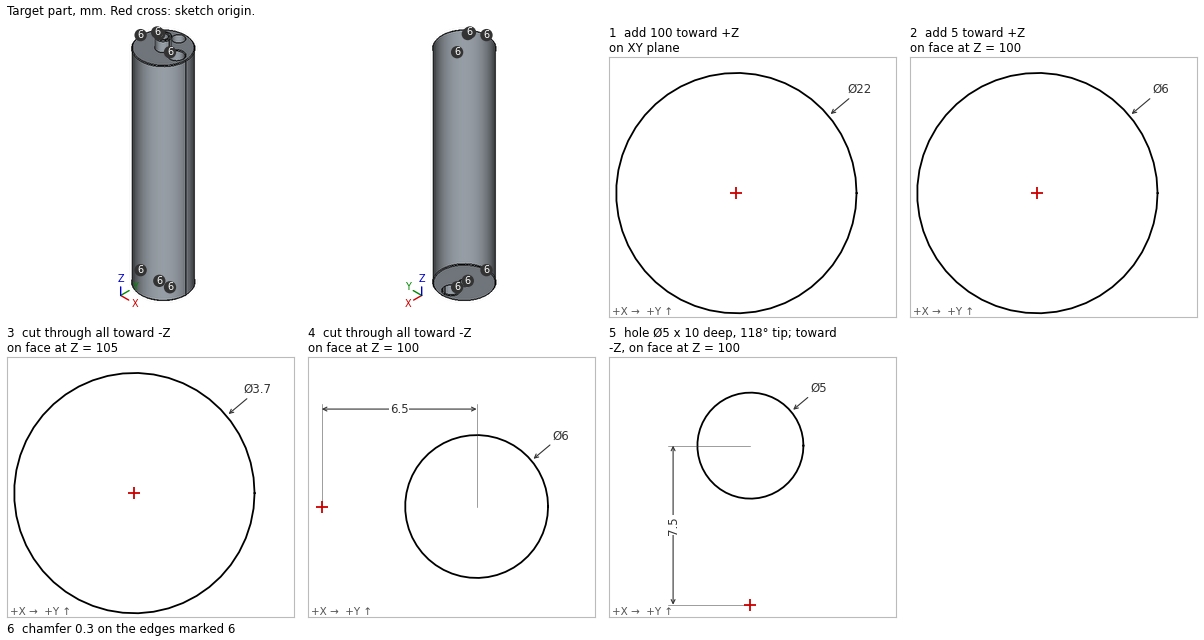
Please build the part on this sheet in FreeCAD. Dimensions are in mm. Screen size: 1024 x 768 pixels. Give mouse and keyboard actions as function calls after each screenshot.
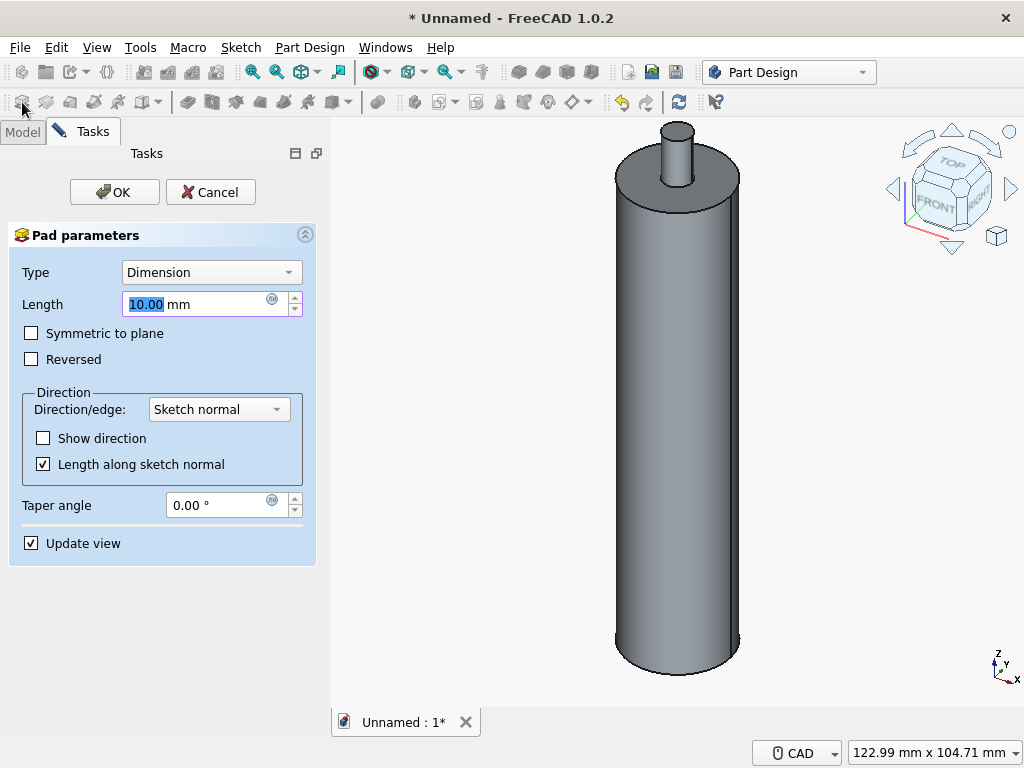
text(5)
key(Tab)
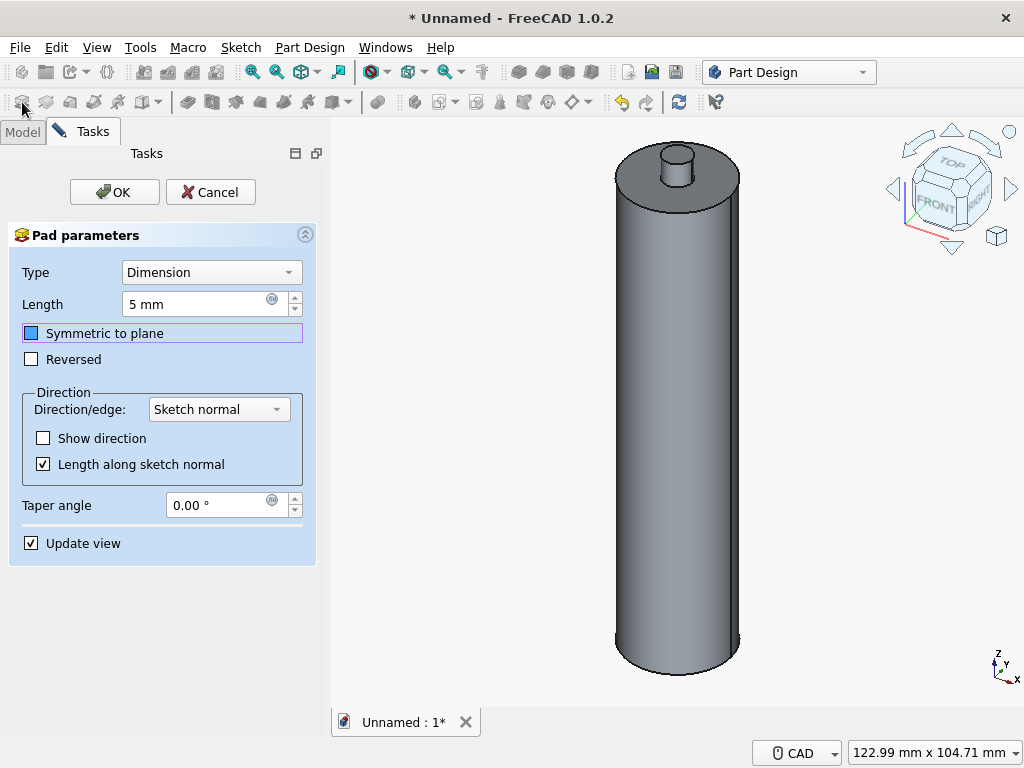
click(115, 192)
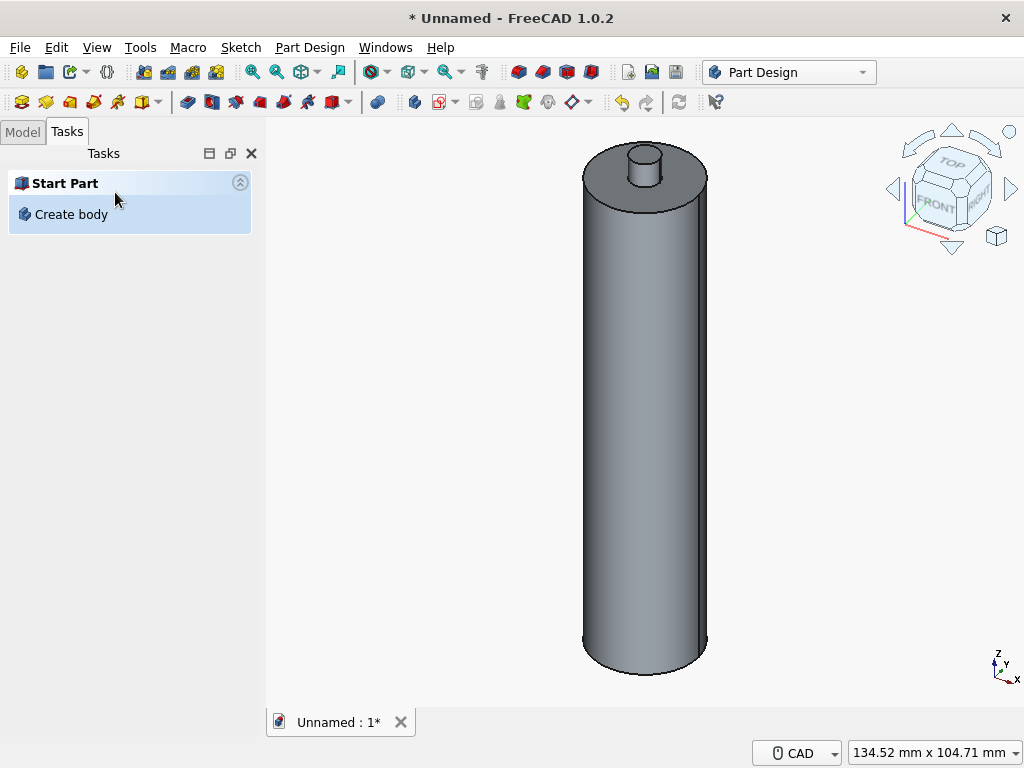
click(254, 72)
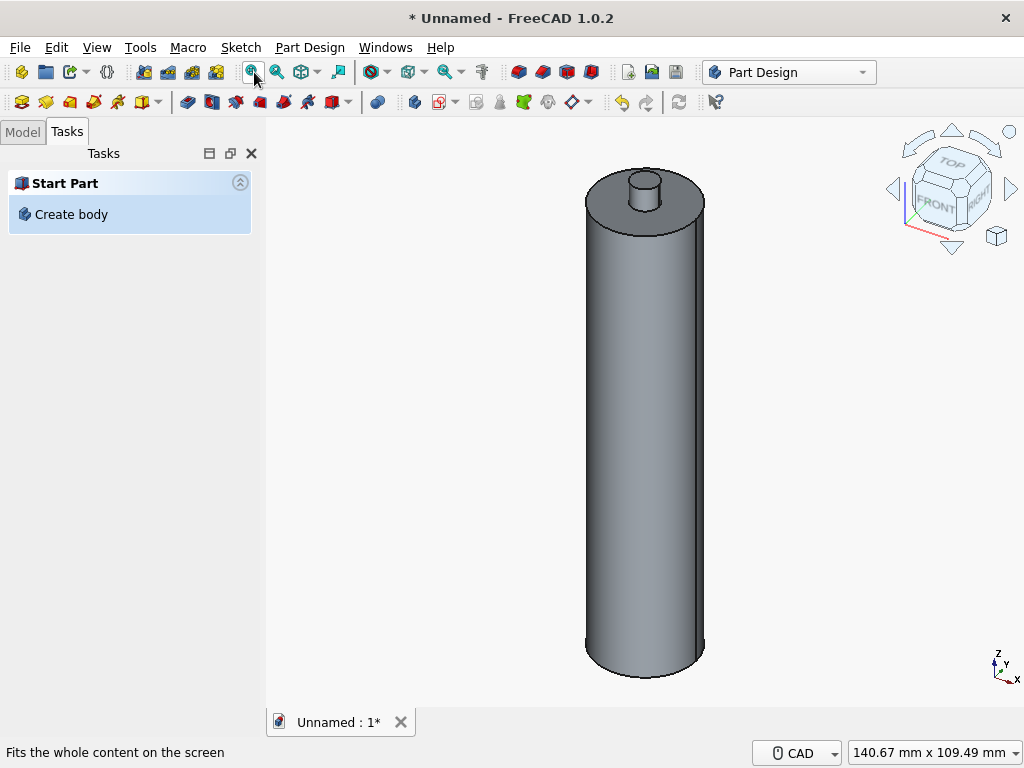
click(645, 179)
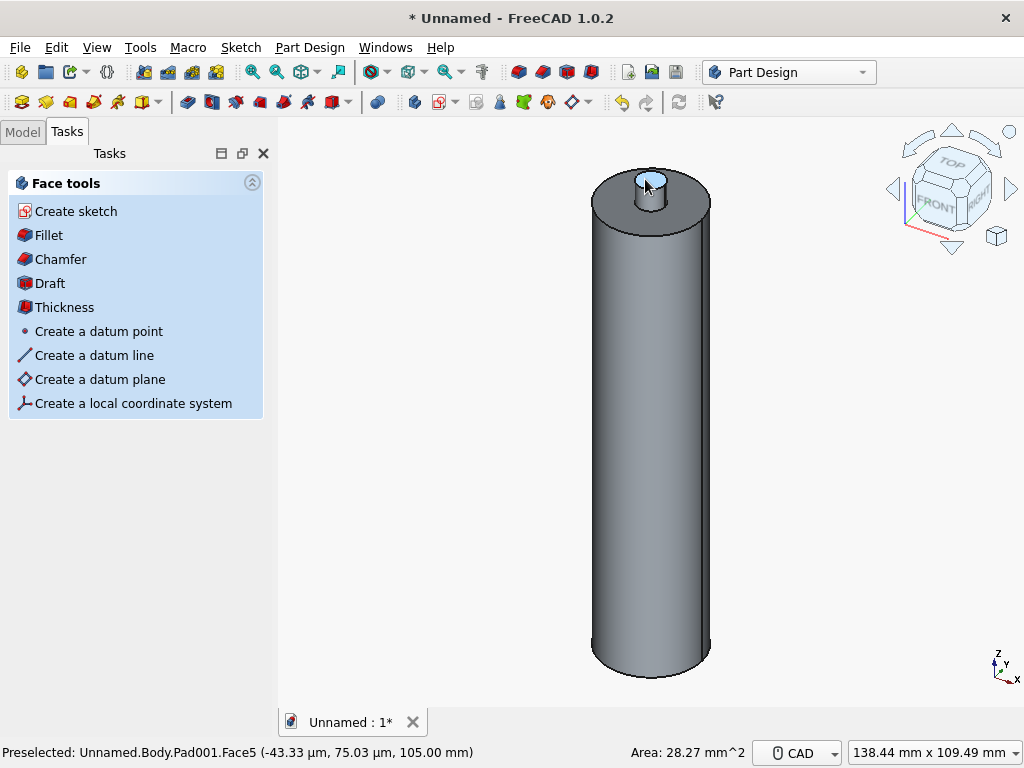
click(440, 102)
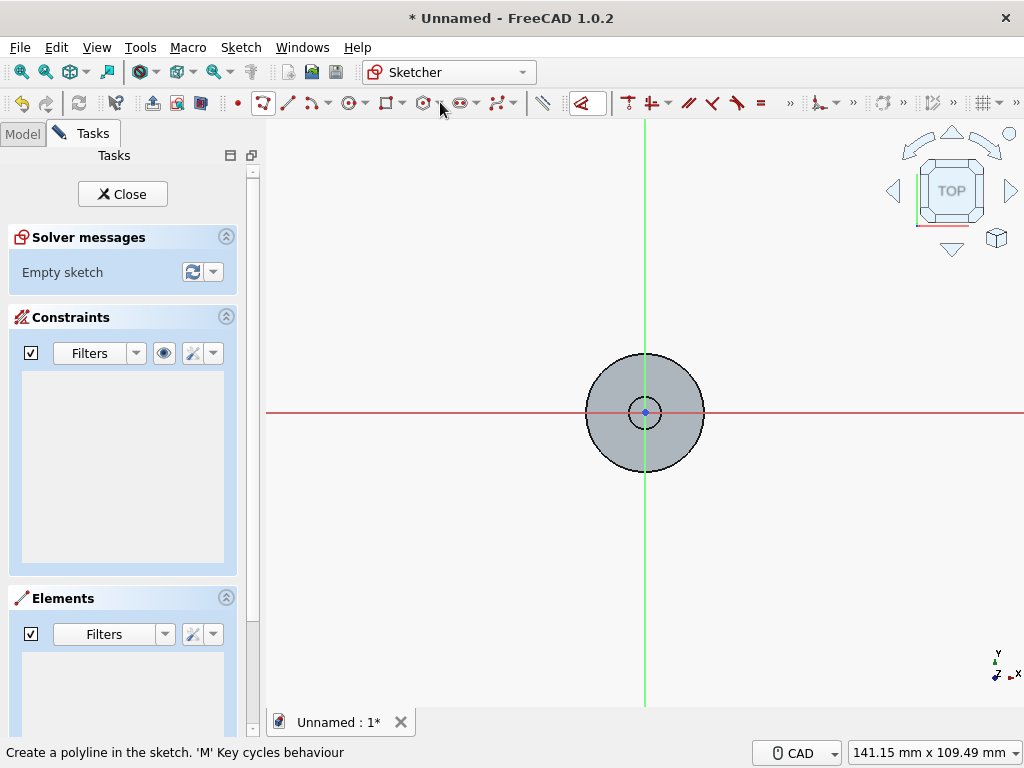
scroll(649, 413, up, 15)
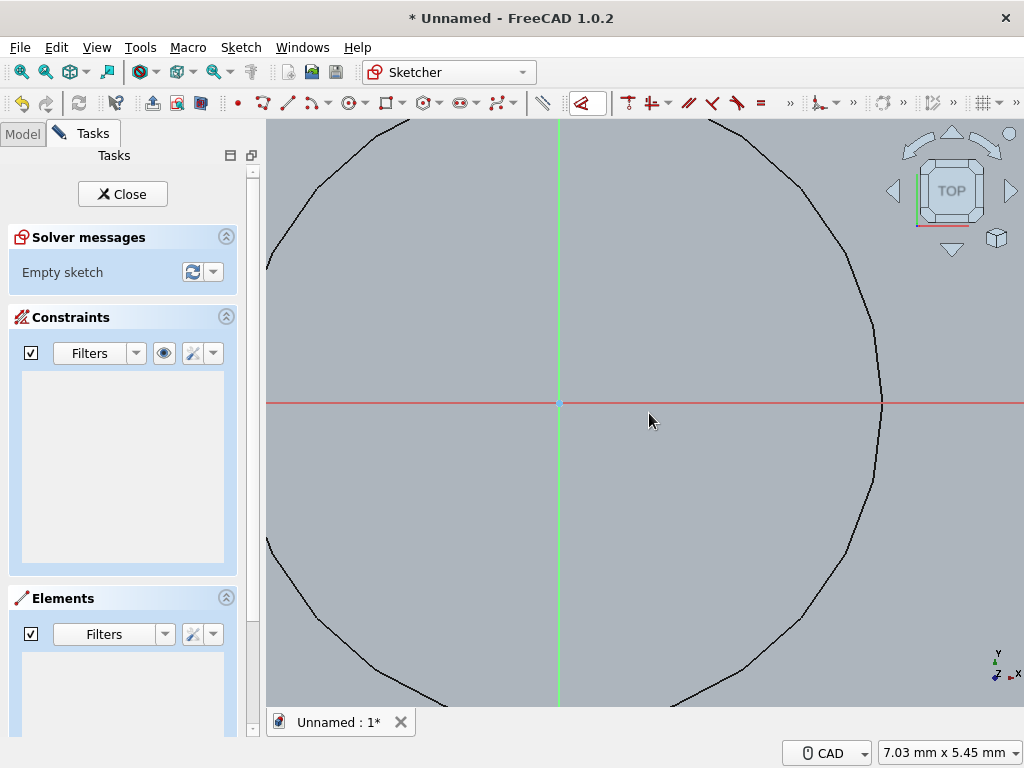
click(350, 104)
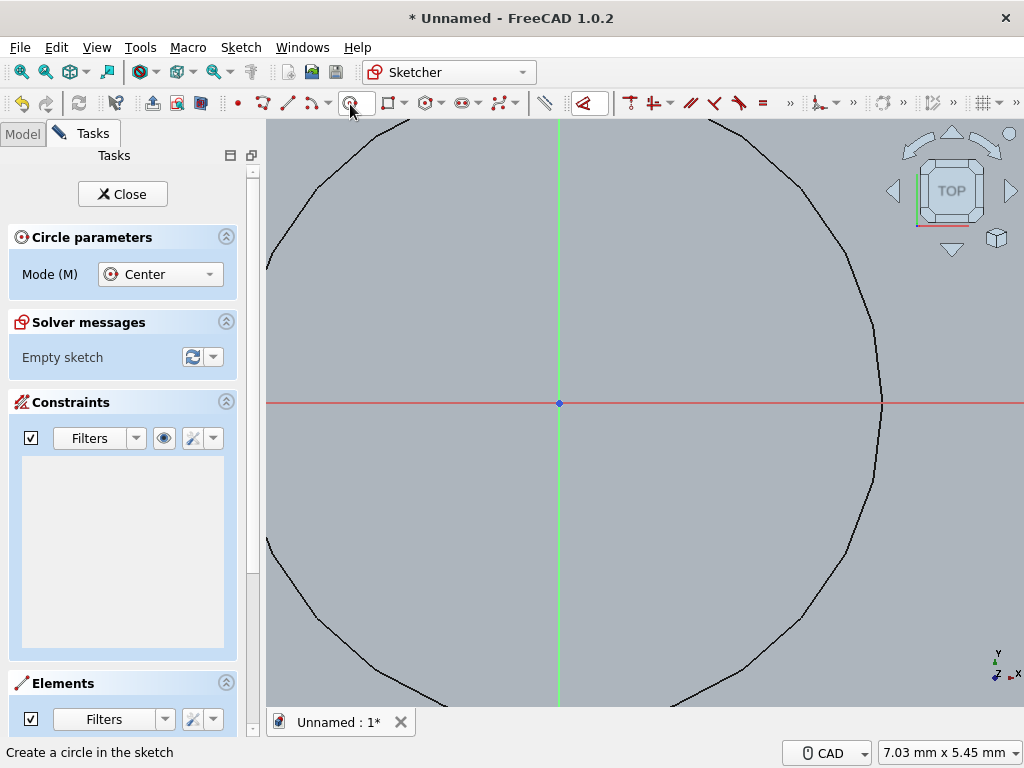
click(559, 403)
click(700, 262)
key(Escape)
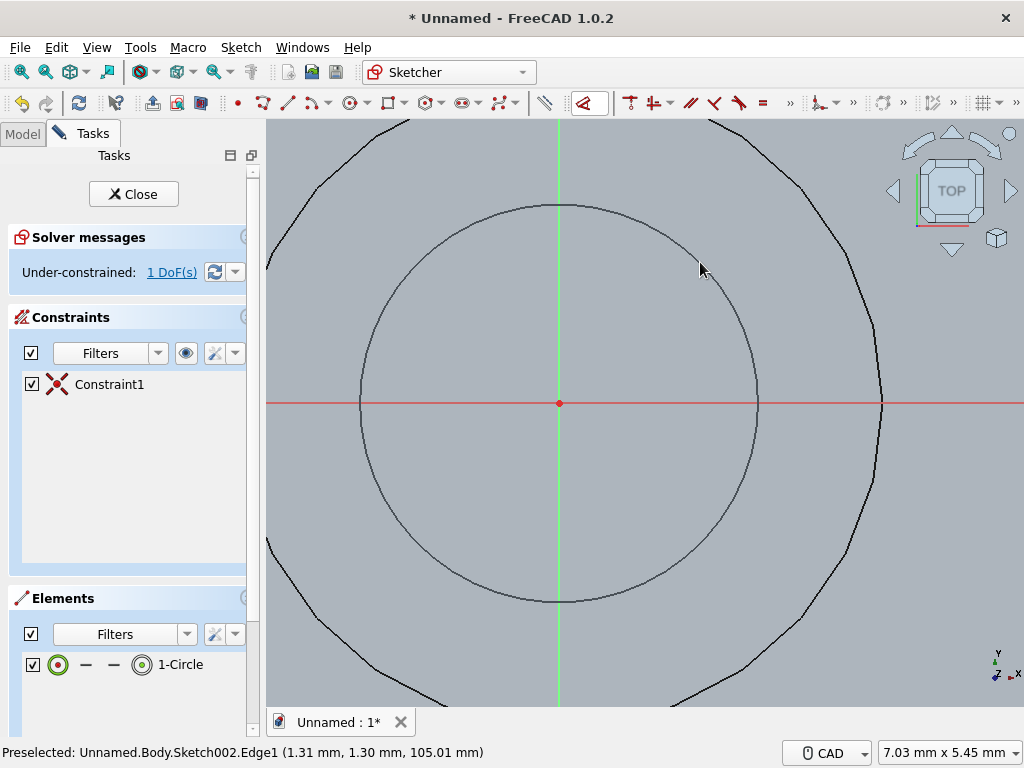
click(699, 262)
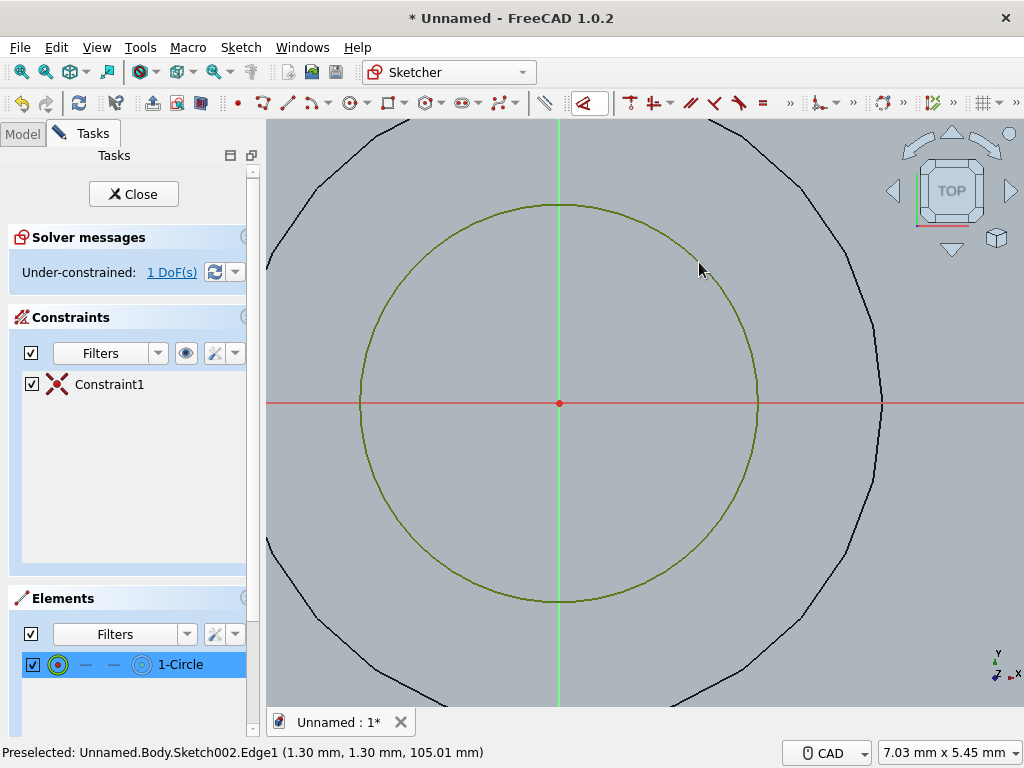
key(k)
key(o)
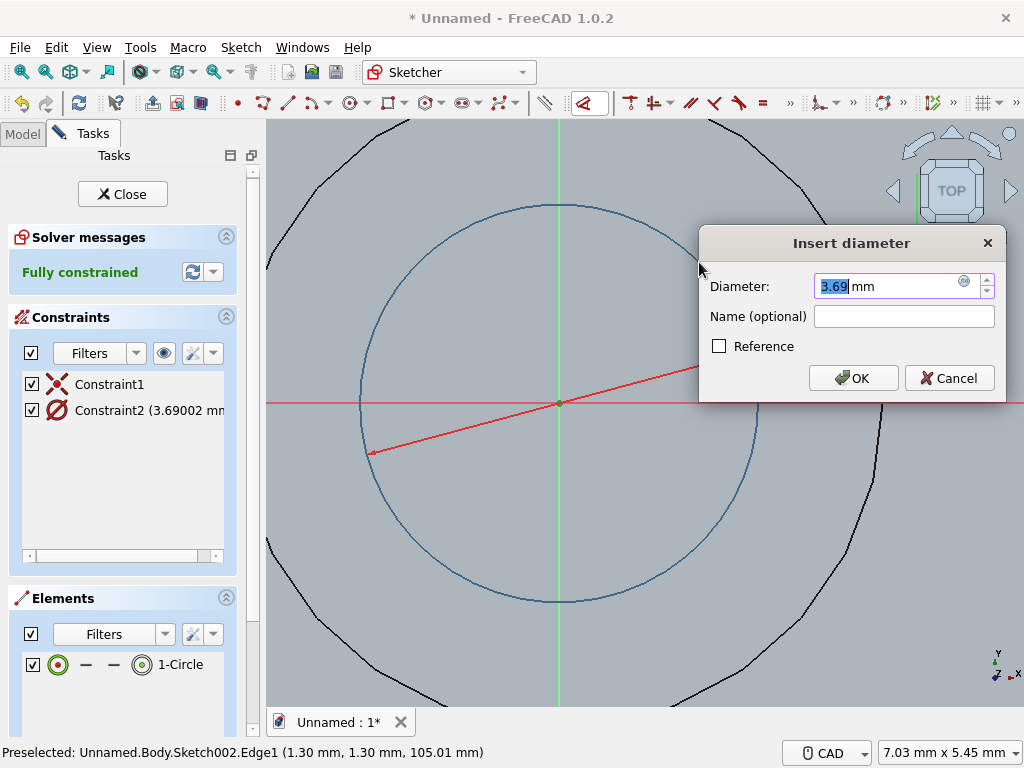
text(3.7)
key(Return)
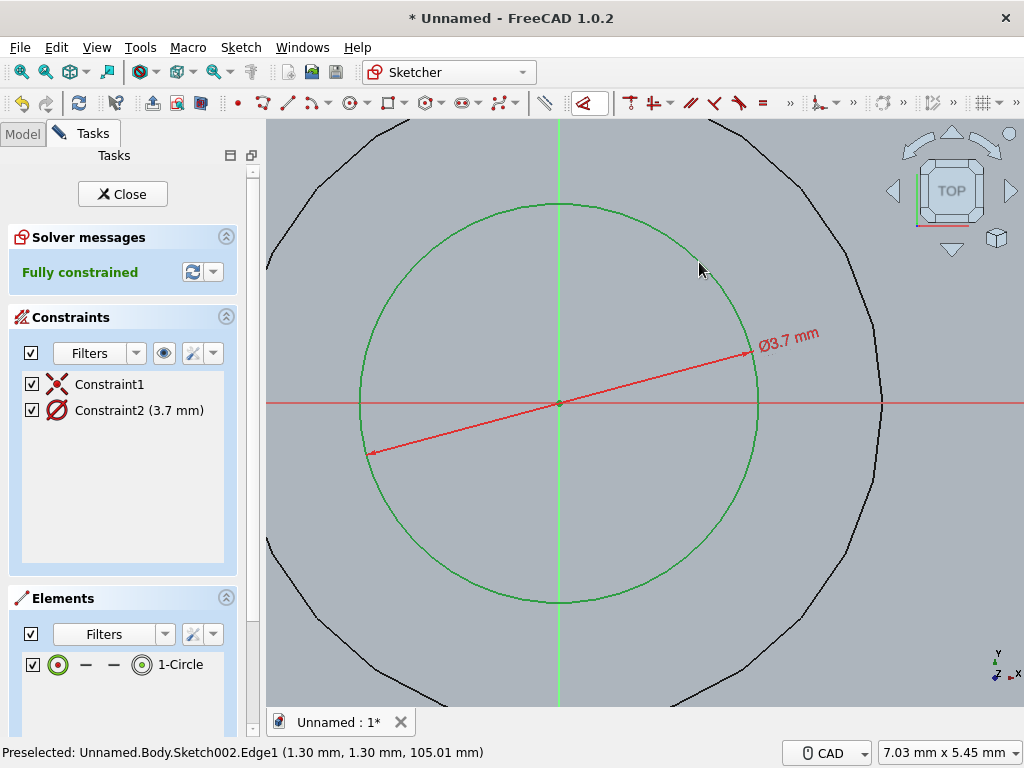
click(123, 194)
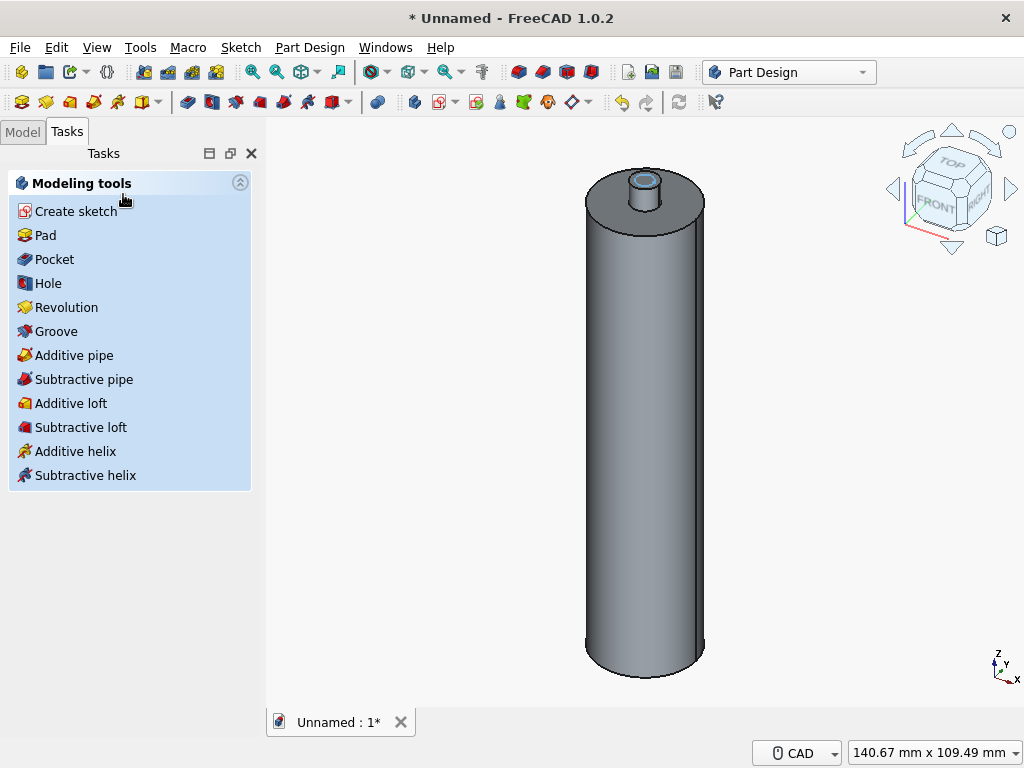
click(188, 102)